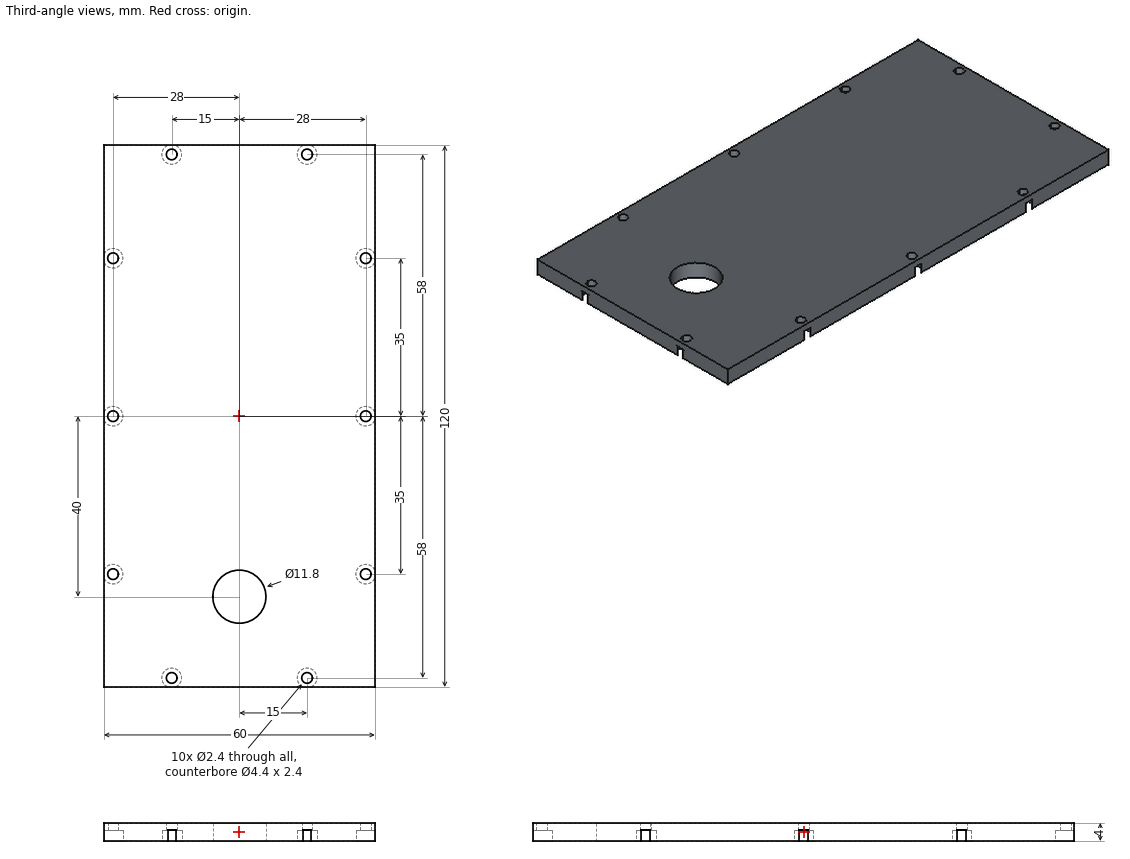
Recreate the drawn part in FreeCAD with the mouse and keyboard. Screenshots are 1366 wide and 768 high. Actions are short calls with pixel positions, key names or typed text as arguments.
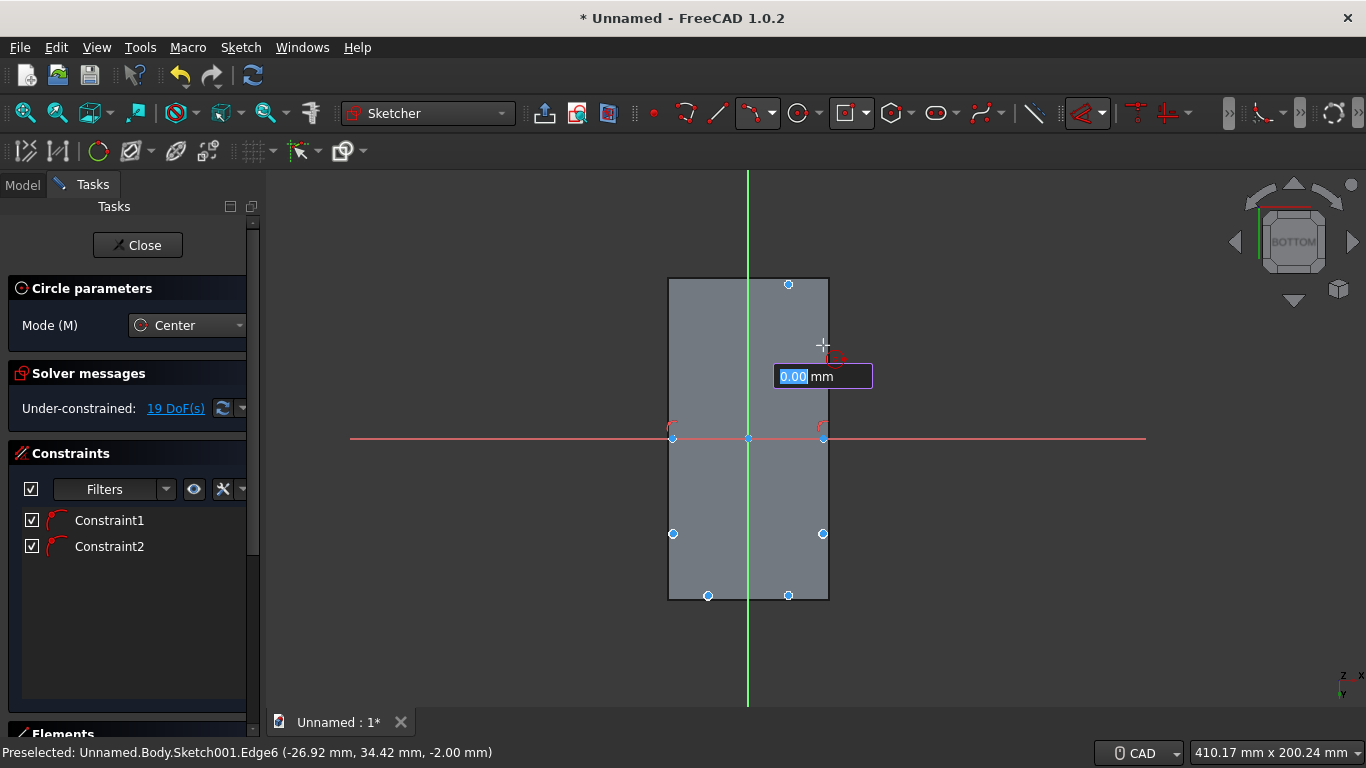
scroll(825, 343, up, 8)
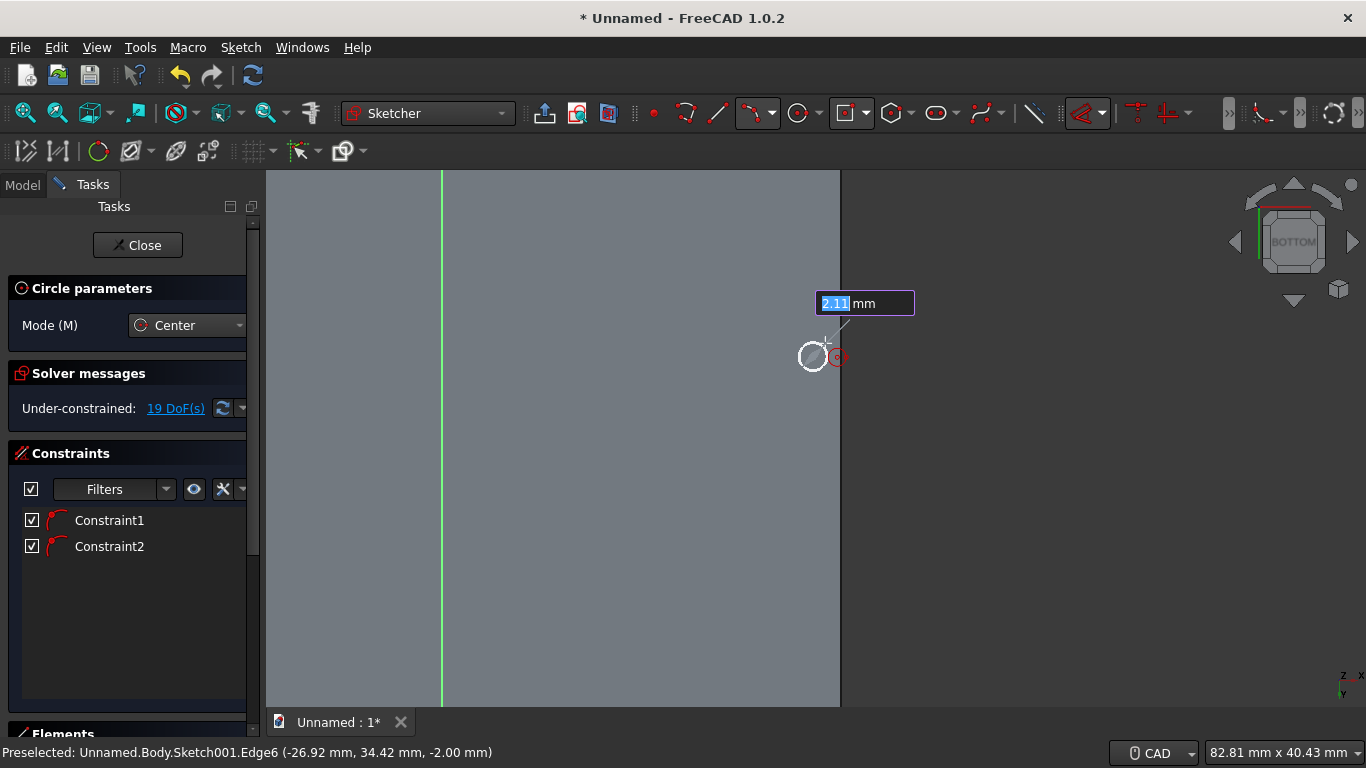
click(825, 341)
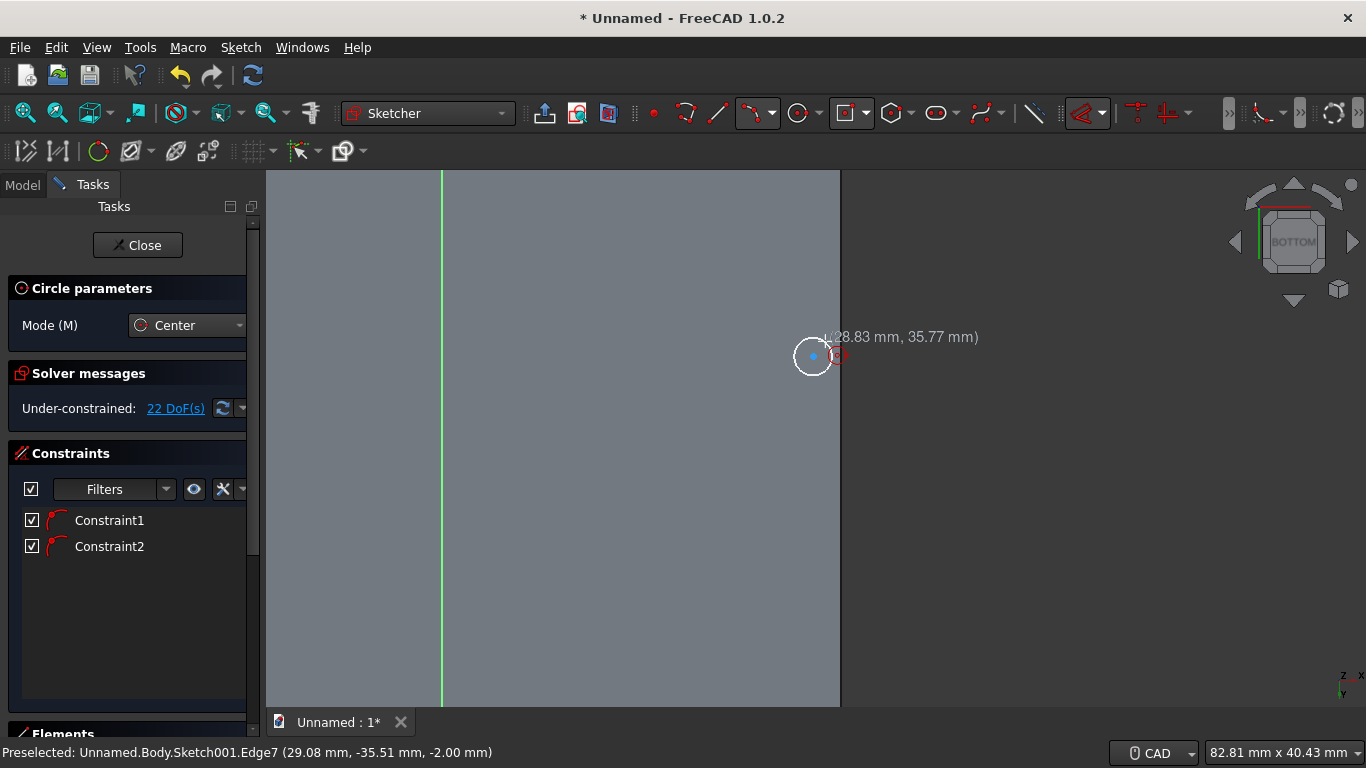
scroll(825, 343, down, 8)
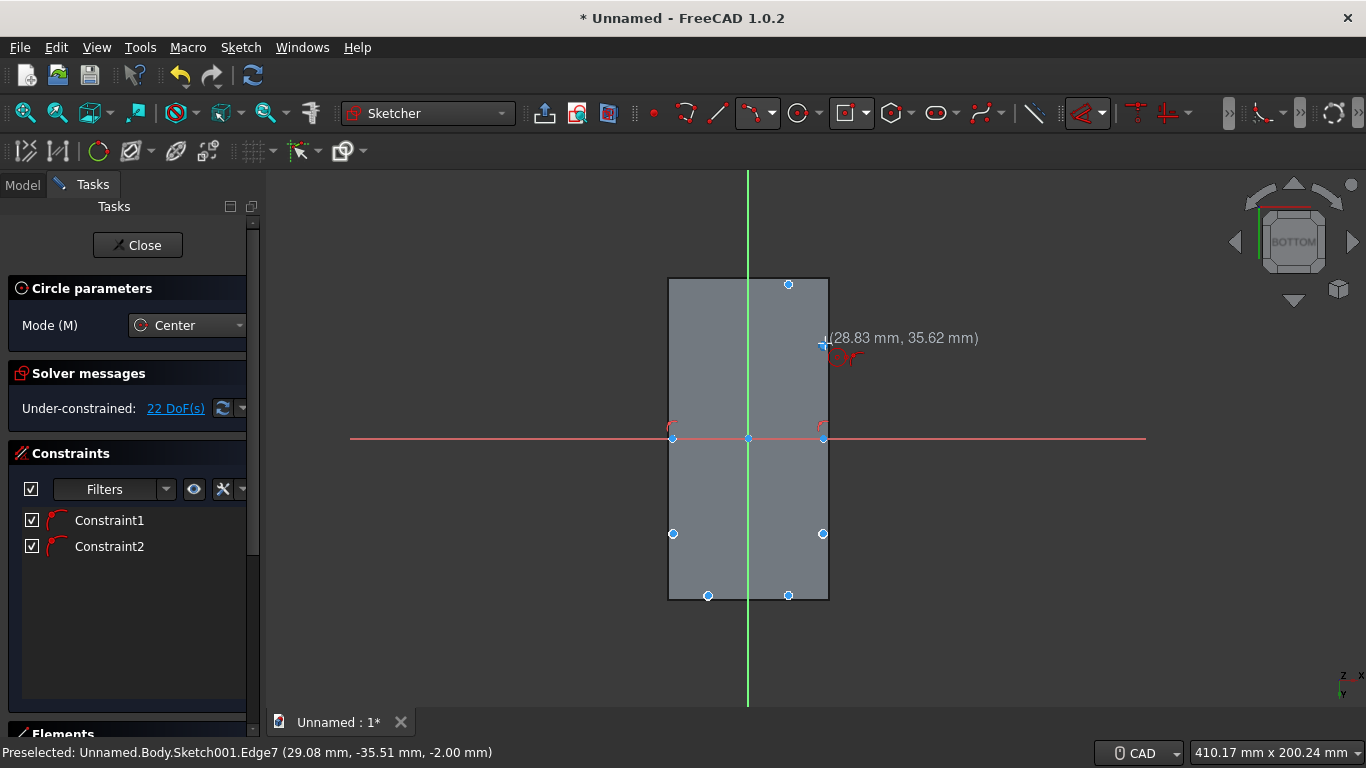
scroll(673, 345, up, 10)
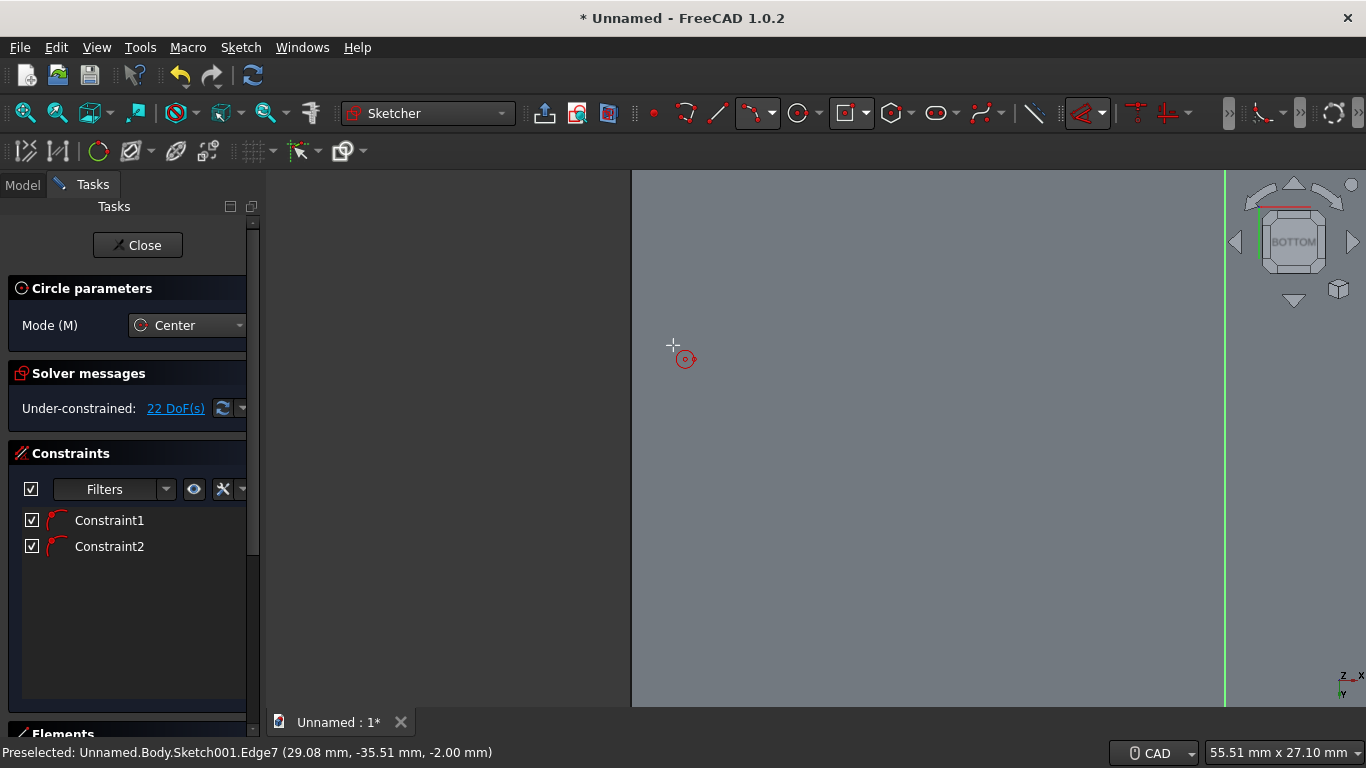
scroll(673, 345, down, 10)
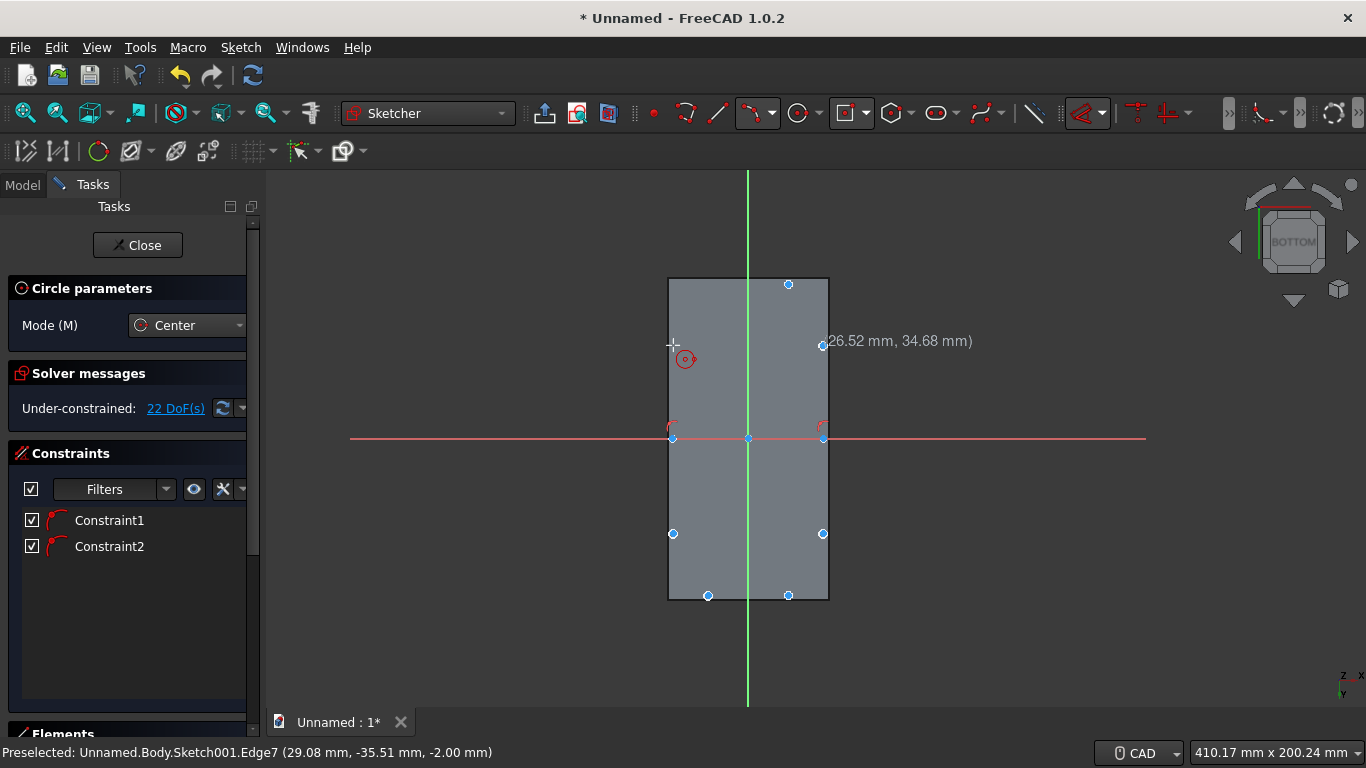
click(673, 345)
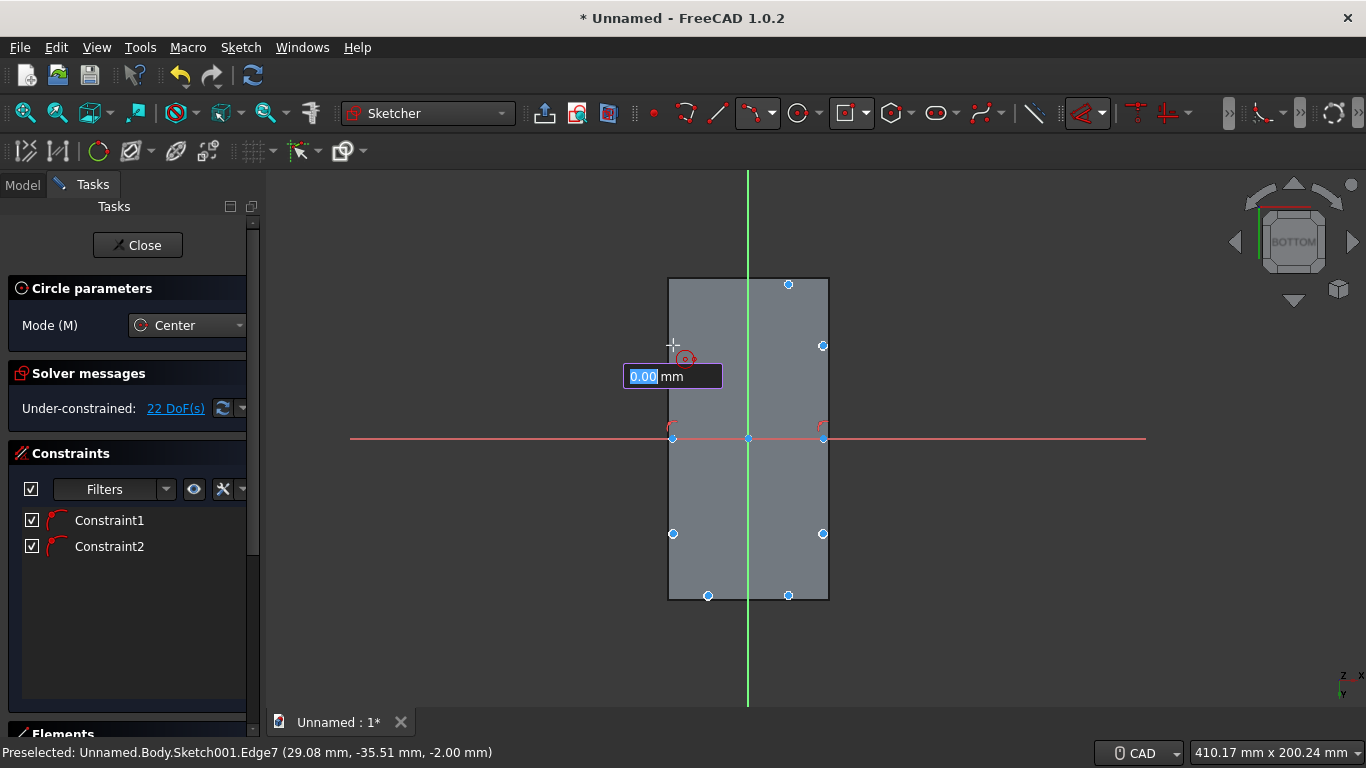
scroll(675, 343, up, 8)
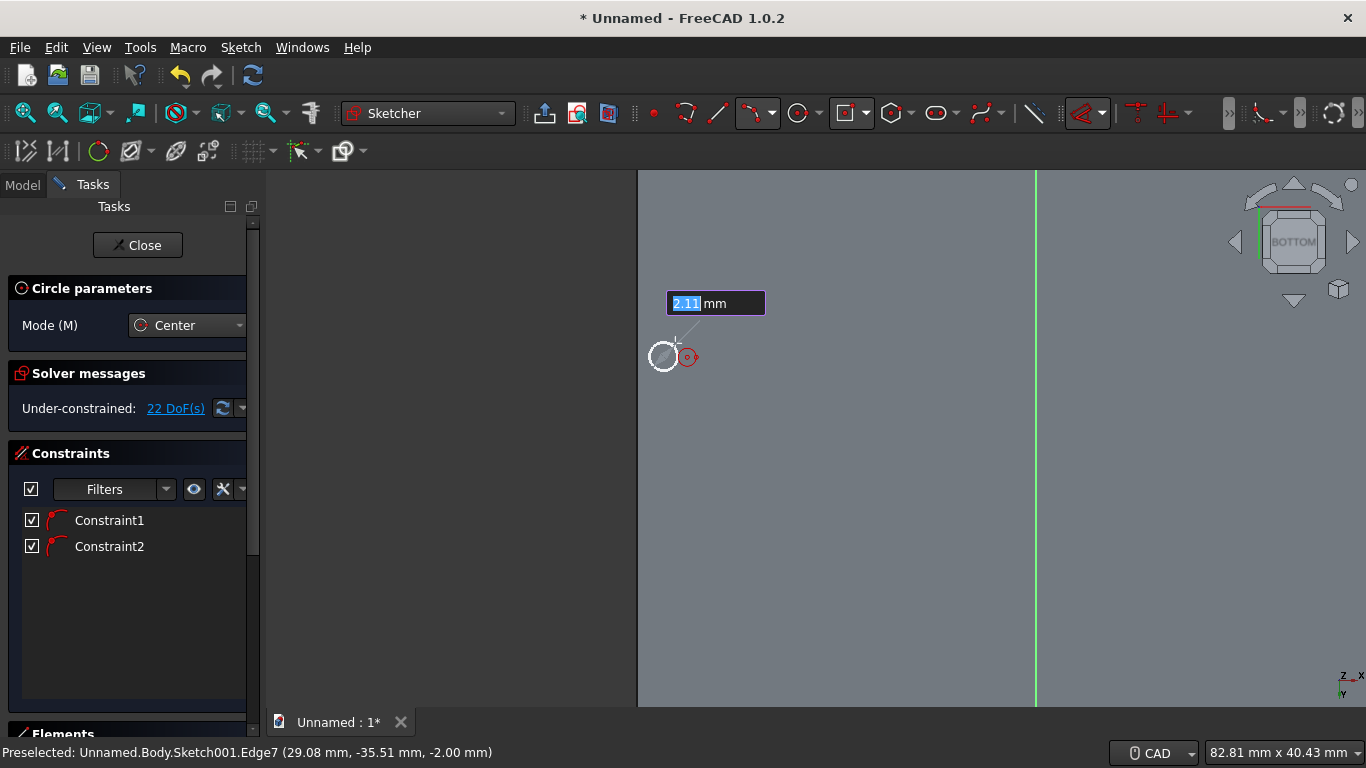
click(675, 341)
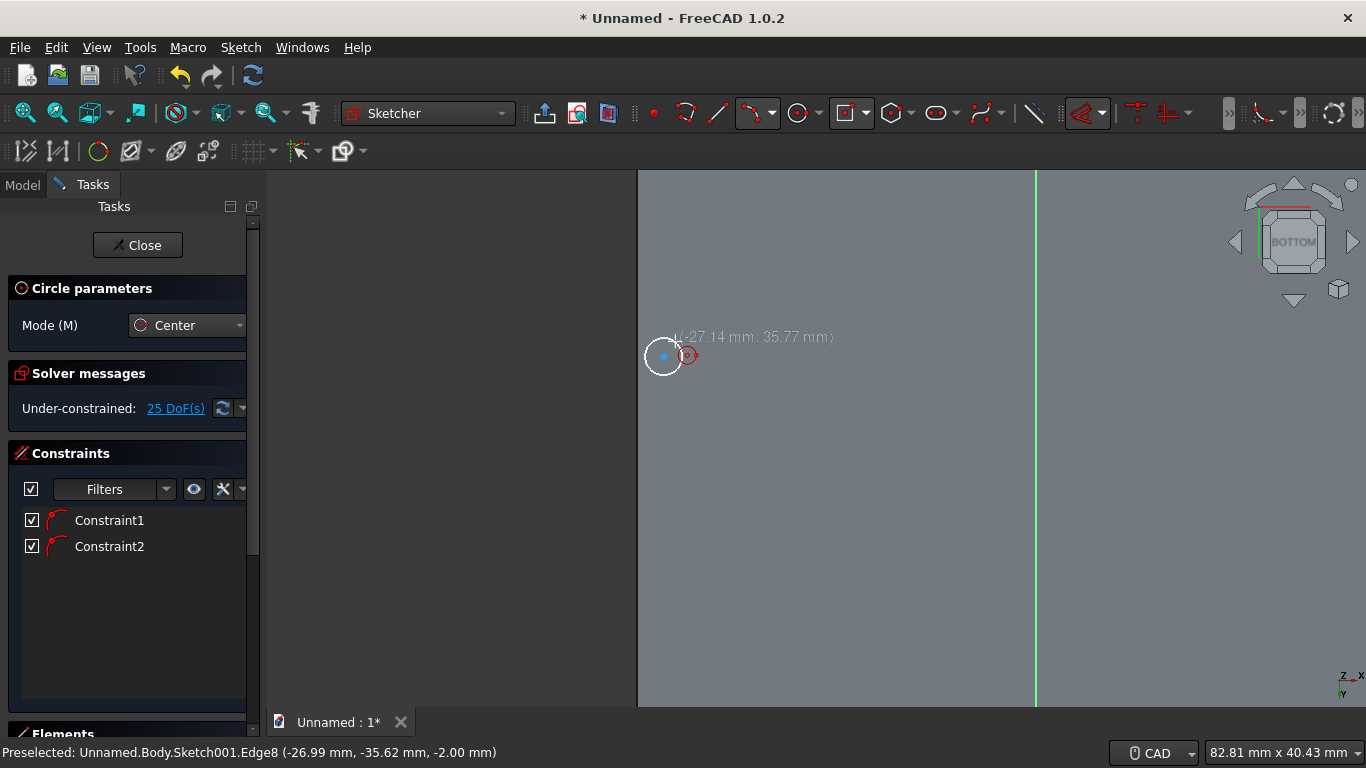
scroll(675, 343, down, 8)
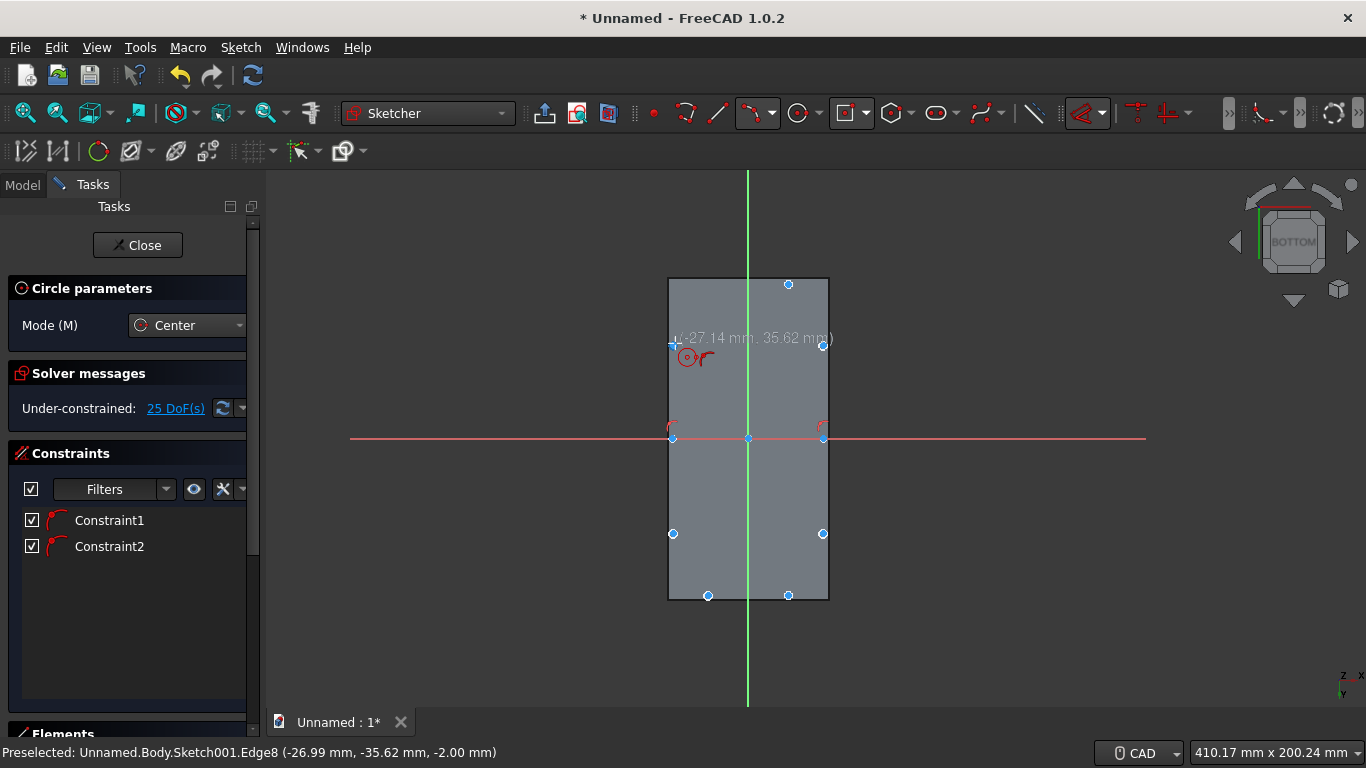
scroll(708, 283, up, 10)